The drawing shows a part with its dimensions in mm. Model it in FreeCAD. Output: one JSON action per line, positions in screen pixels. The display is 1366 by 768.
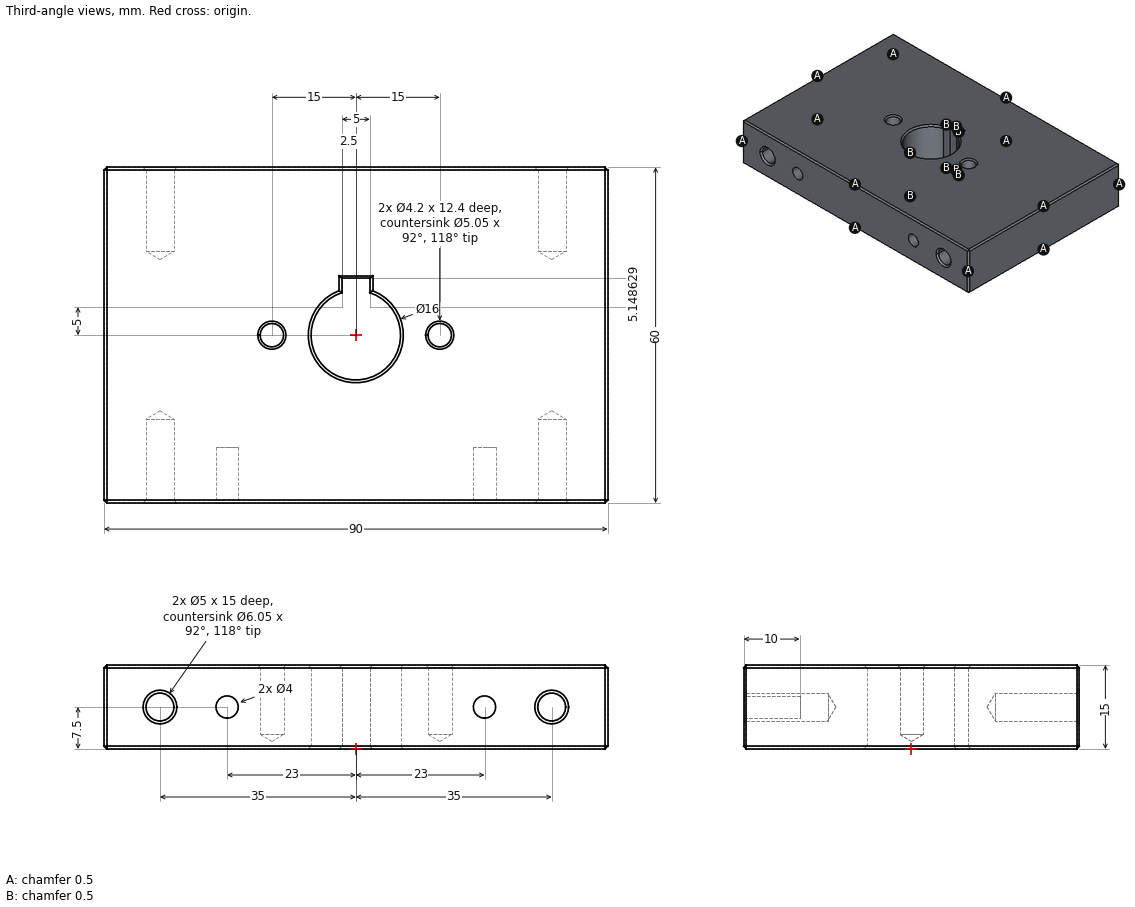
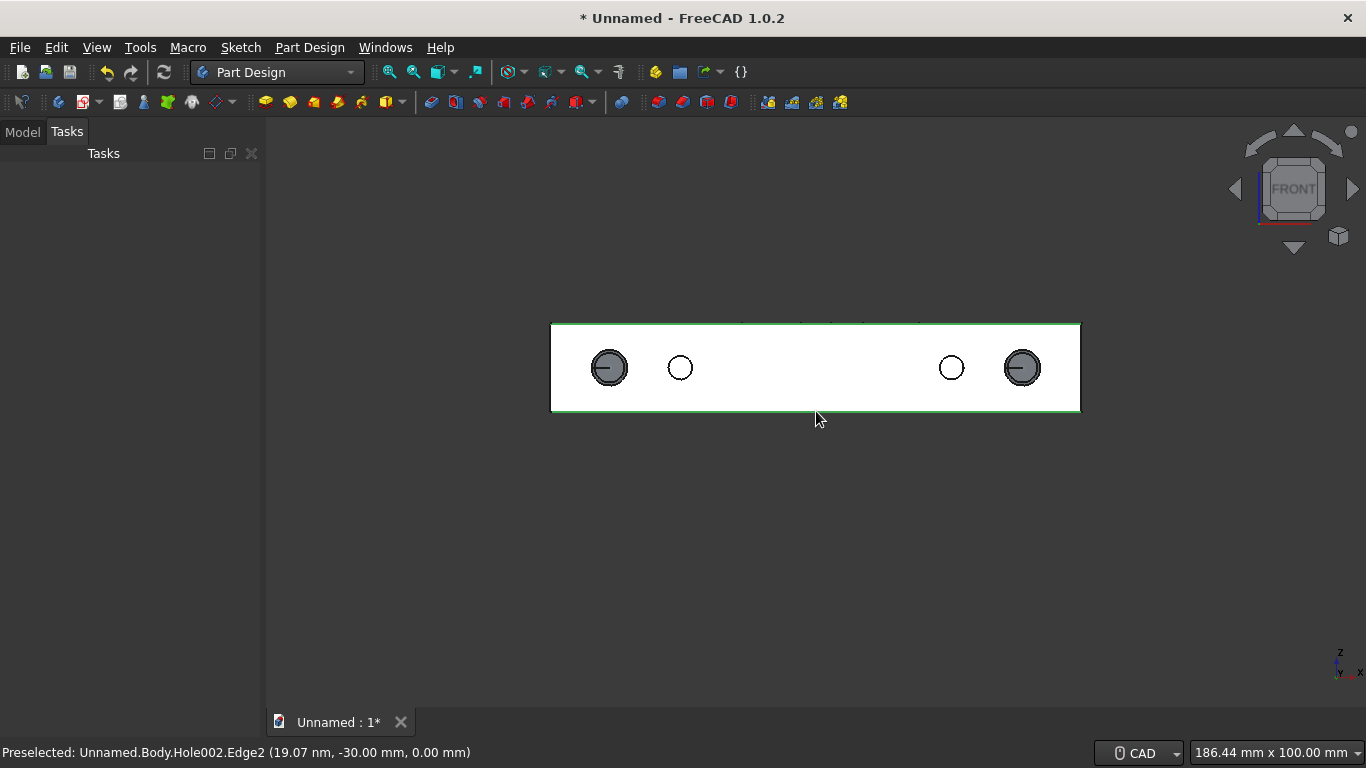
{"action": "key", "text": "3"}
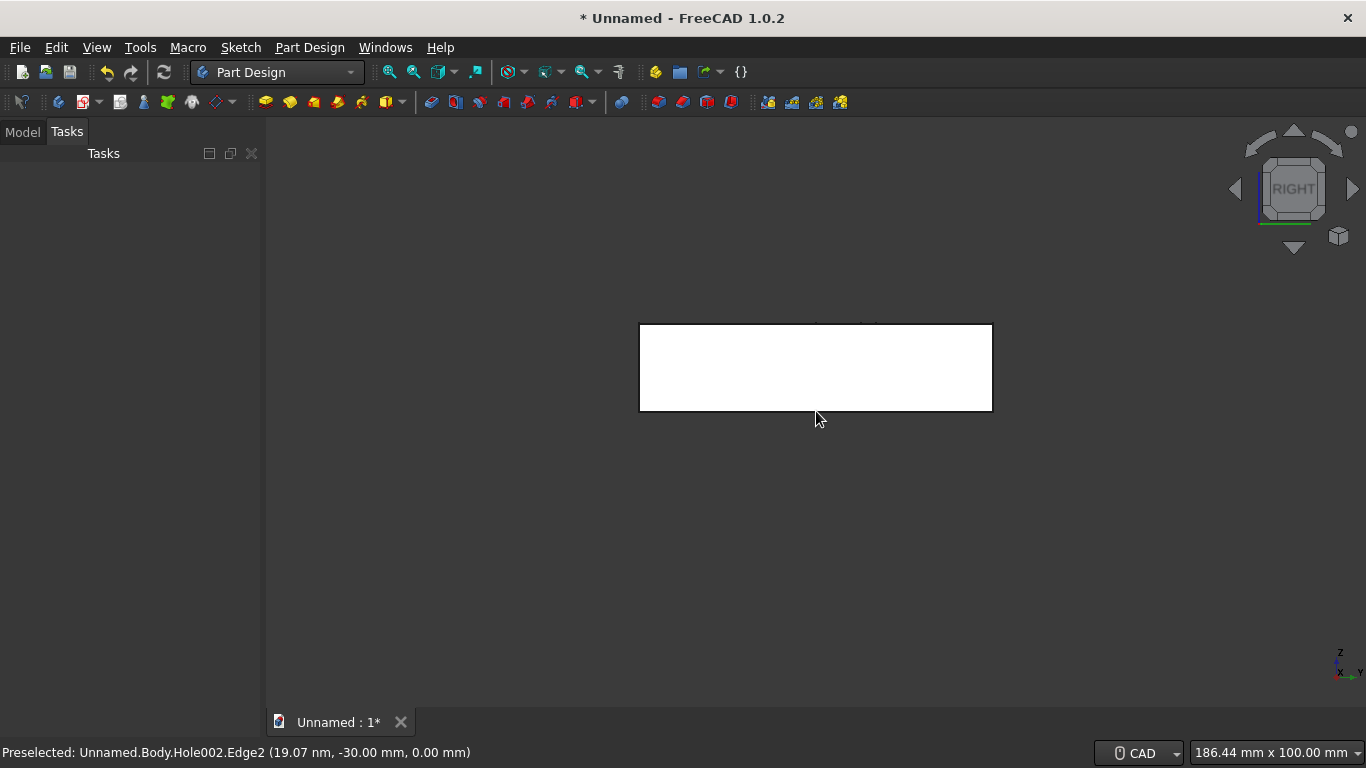
{"action": "left_click", "coordinate": [390, 72]}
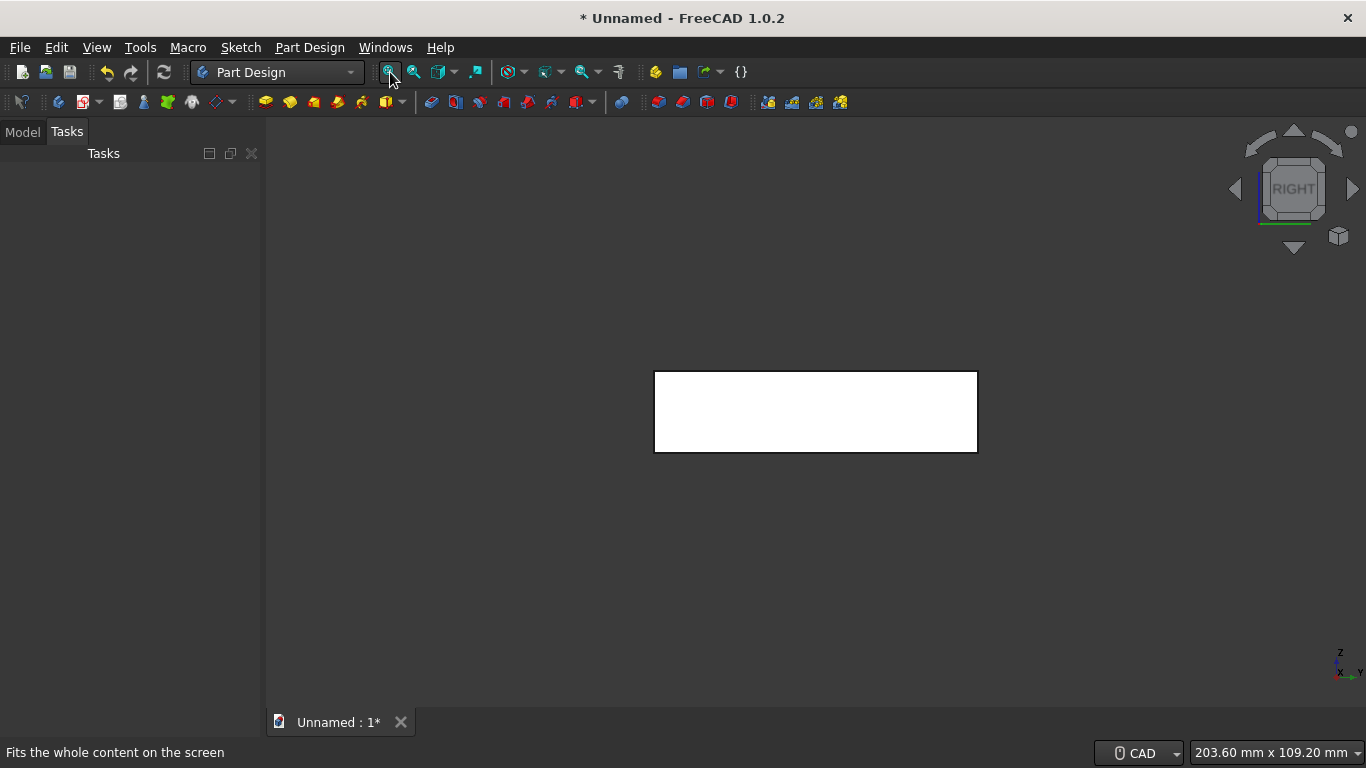
{"action": "key", "text": "5"}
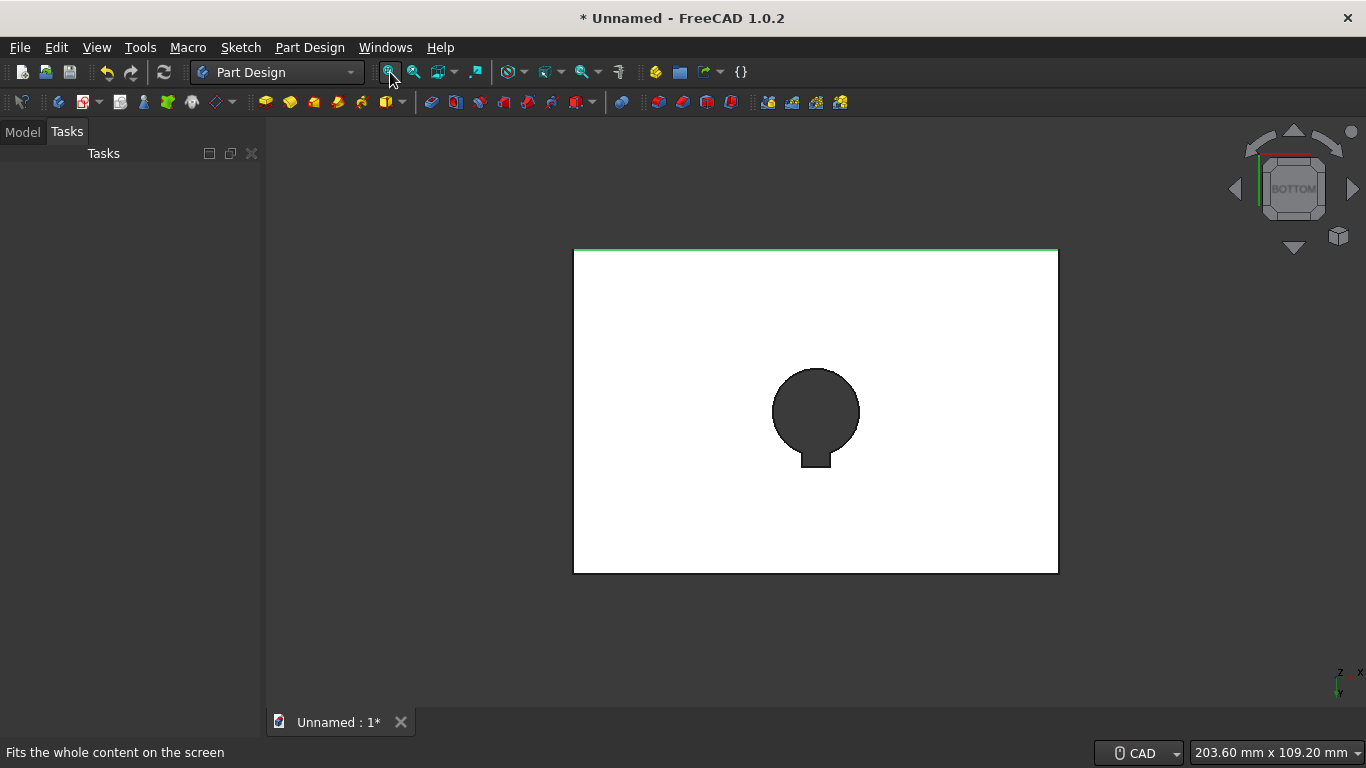
{"action": "left_click", "coordinate": [816, 573], "text": "ctrl"}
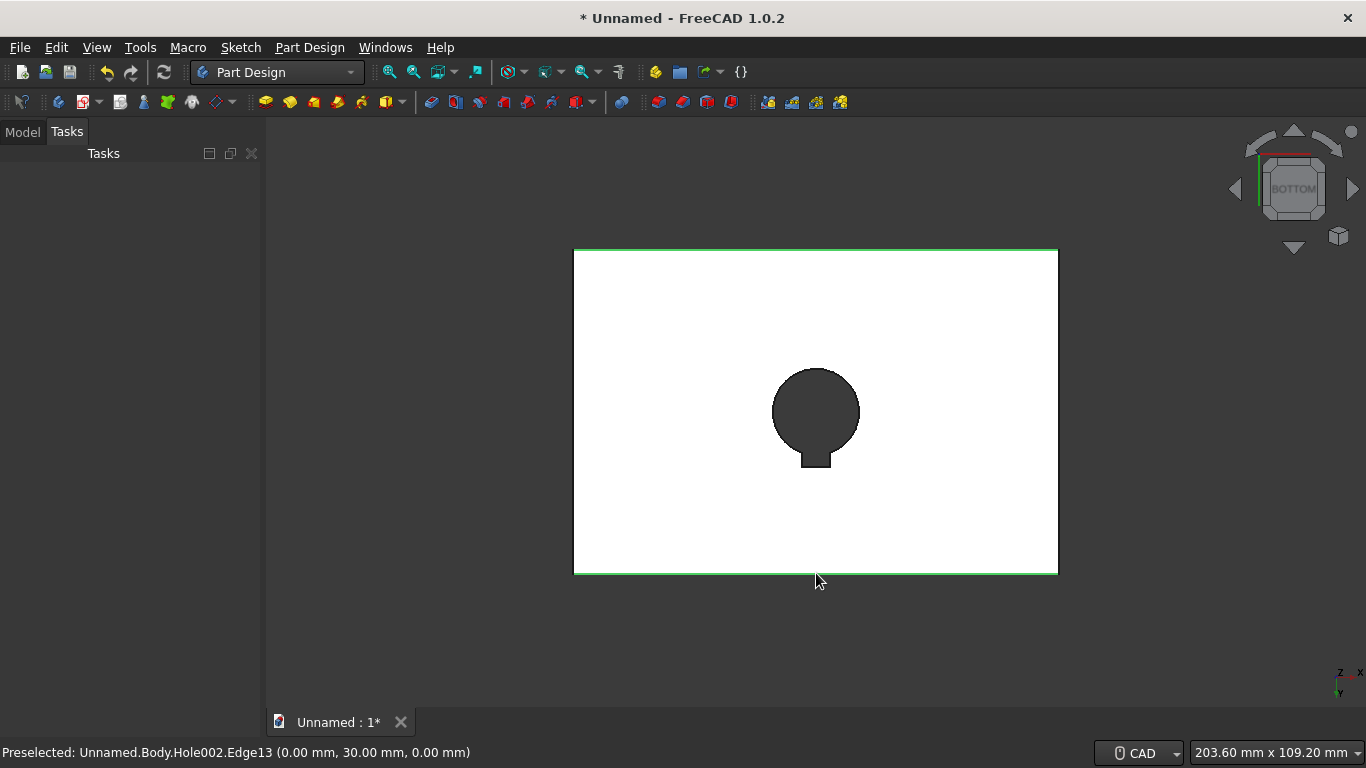
{"action": "key", "text": "4"}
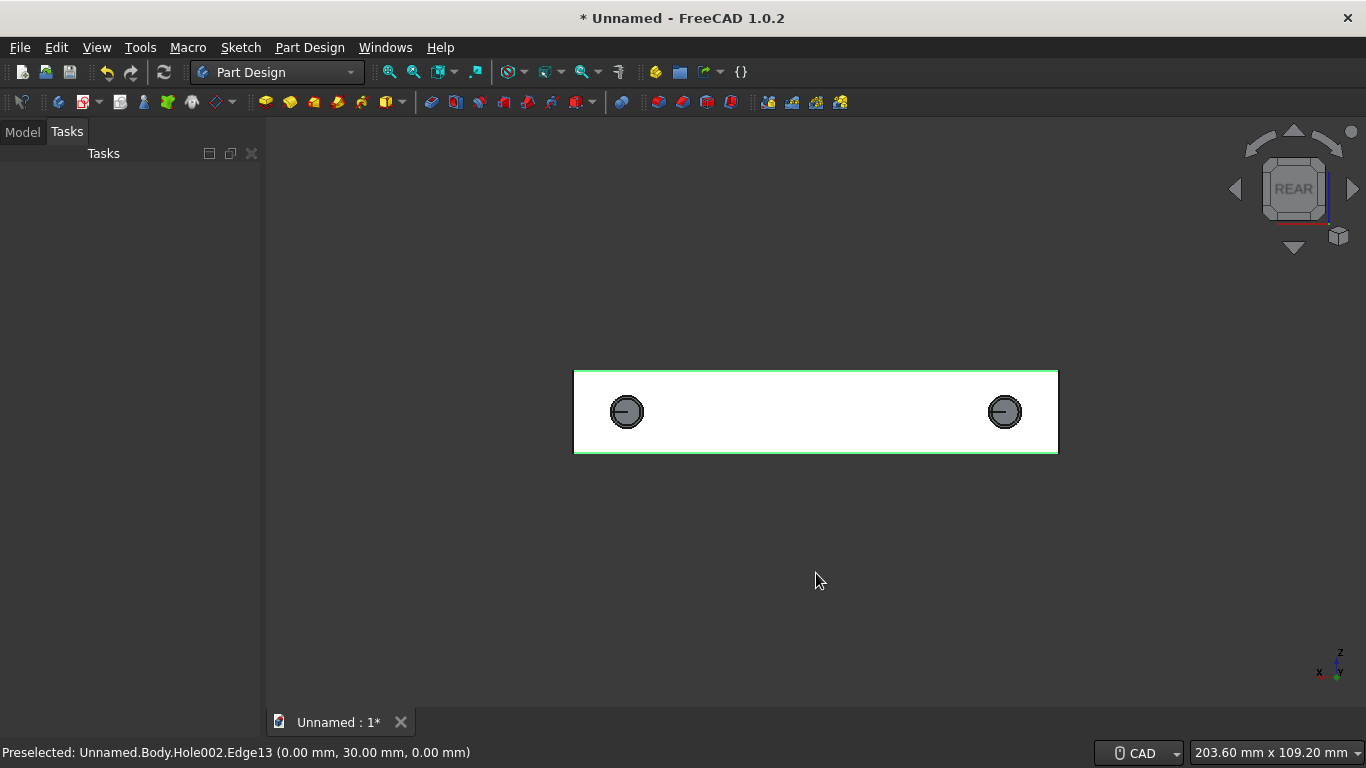
{"action": "left_click", "coordinate": [390, 72]}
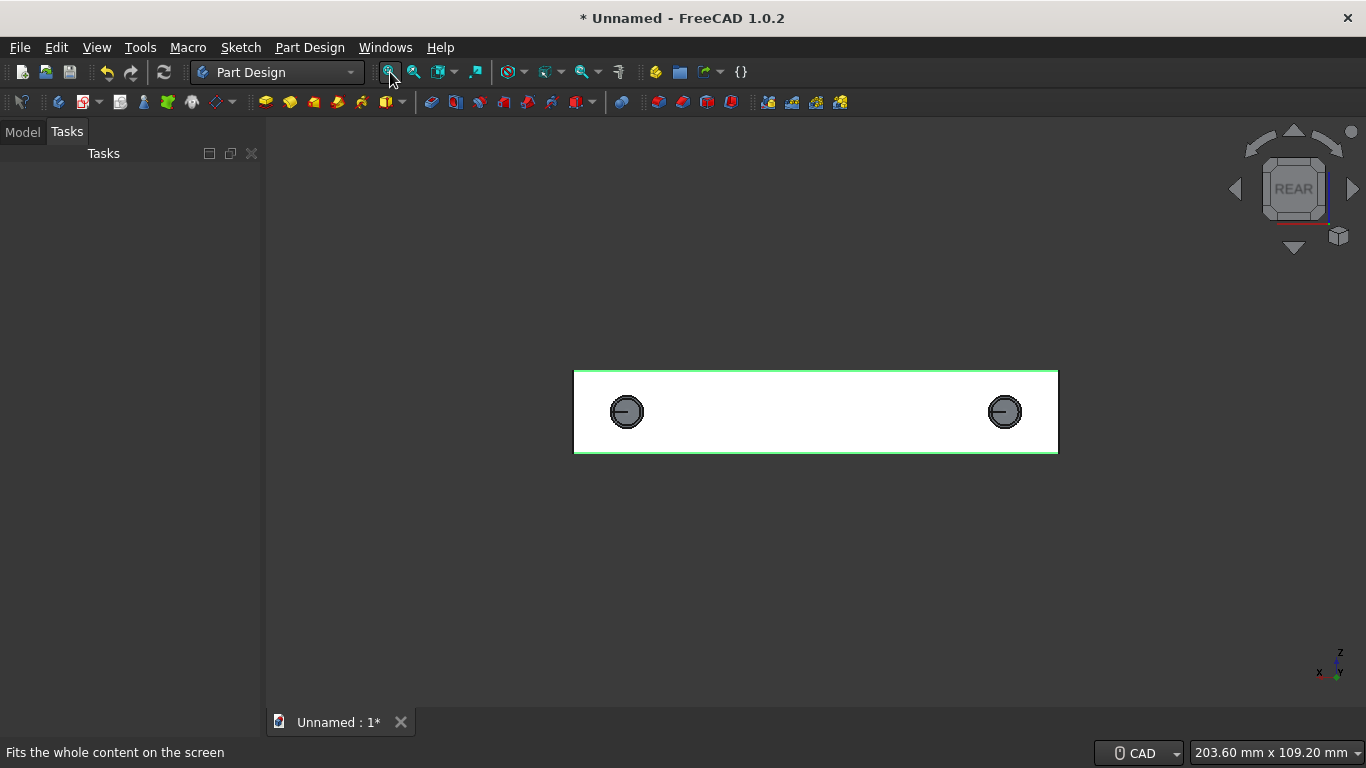
{"action": "key", "text": "6"}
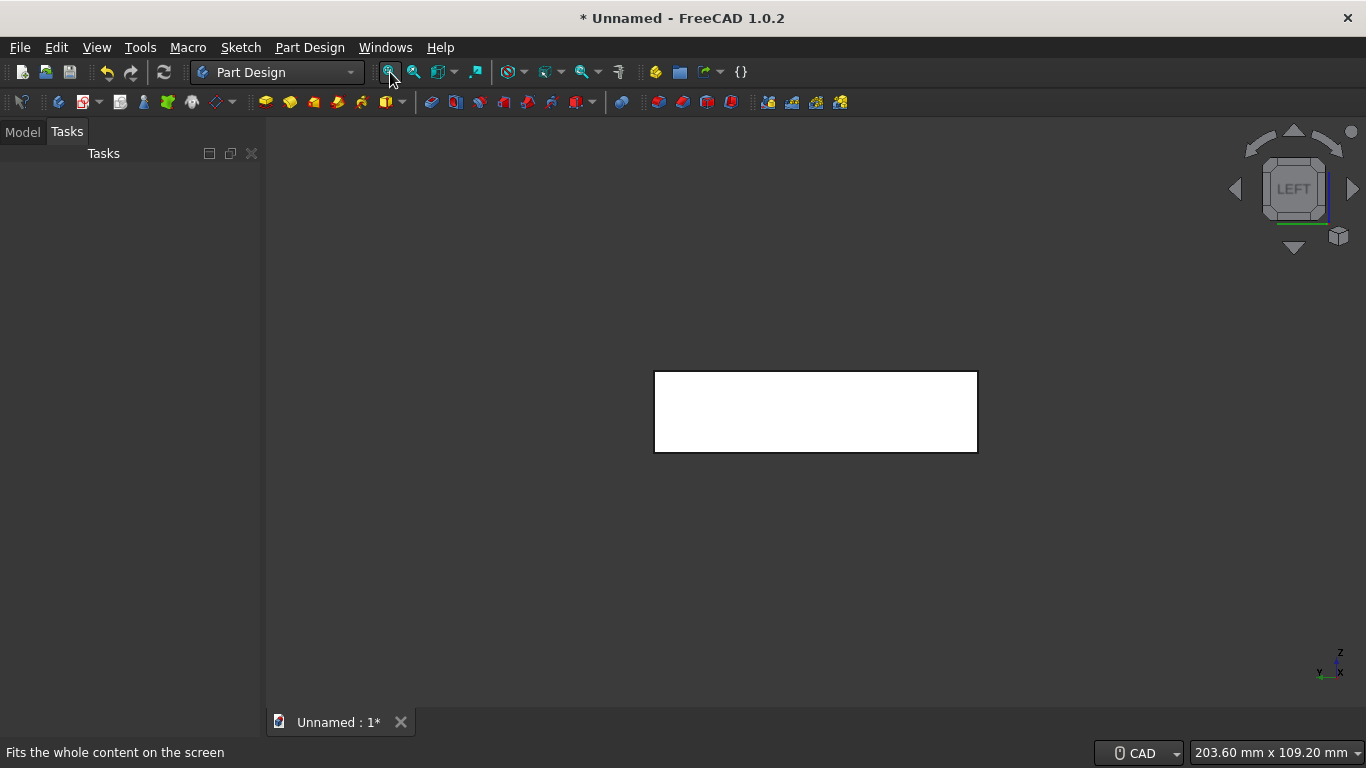
{"action": "key", "text": "v f"}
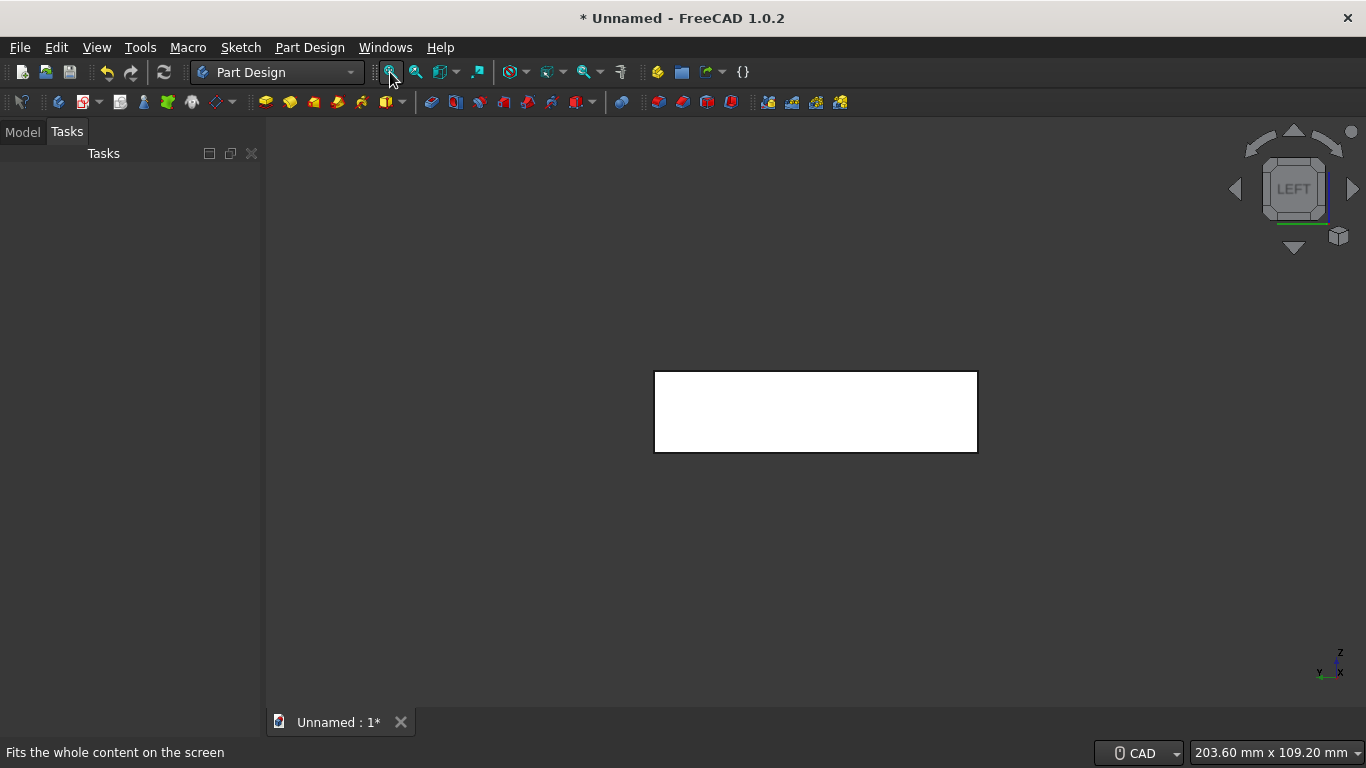
{"action": "left_click", "coordinate": [723, 411], "text": "ctrl"}